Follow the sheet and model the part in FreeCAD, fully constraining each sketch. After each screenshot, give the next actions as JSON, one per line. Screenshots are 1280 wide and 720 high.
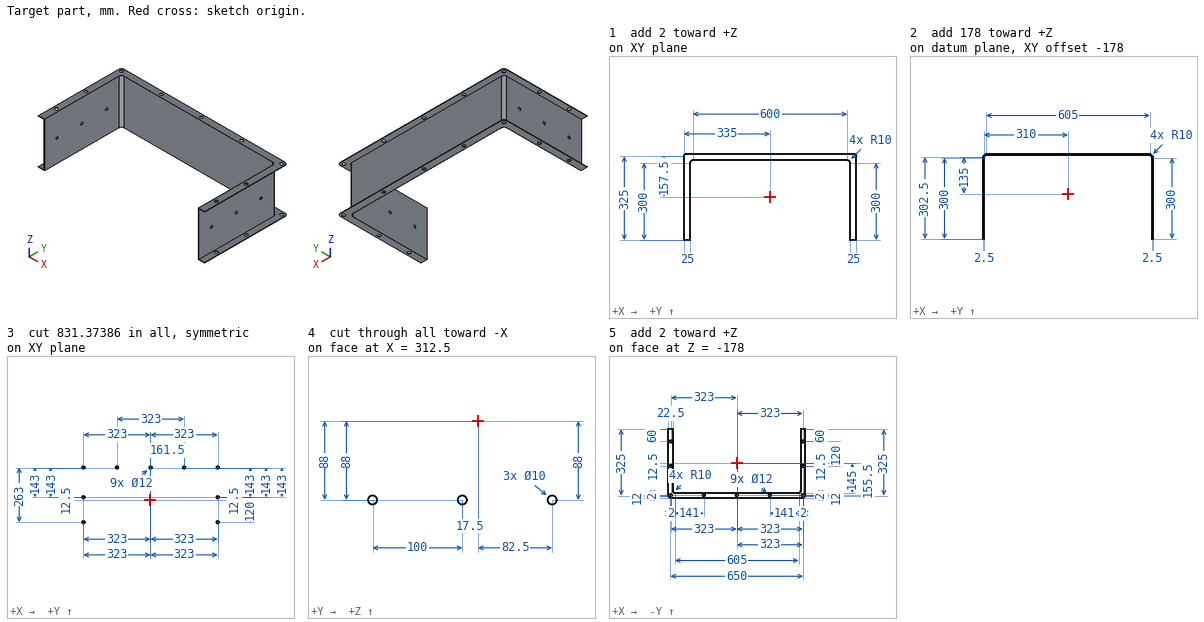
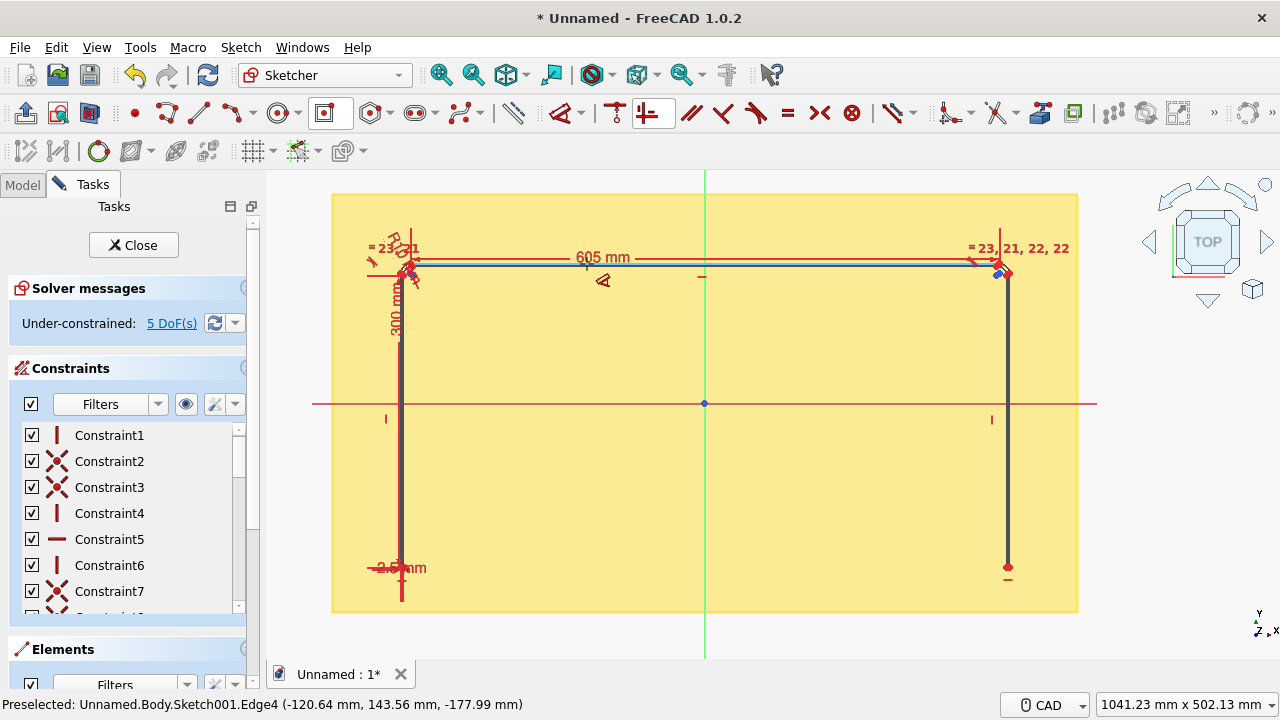
{"action": "scroll", "coordinate": [1008, 568], "scroll_direction": "up", "scroll_amount": 14}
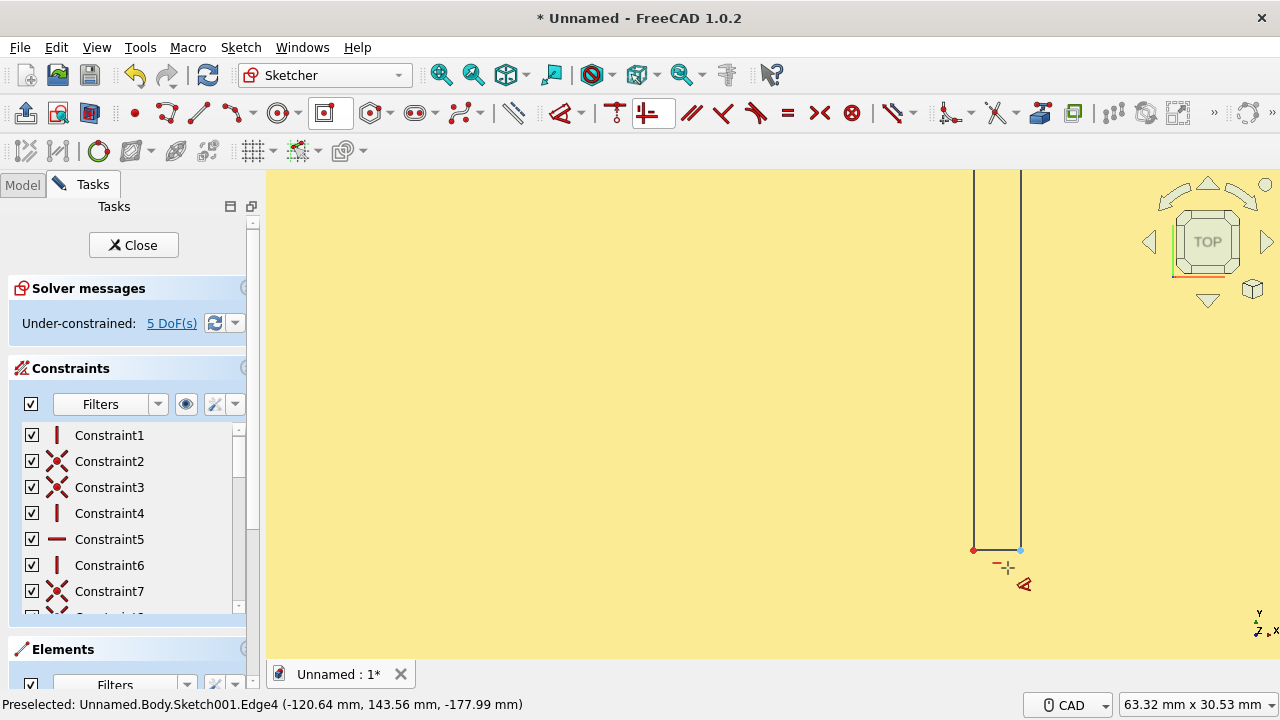
{"action": "left_click", "coordinate": [997, 550]}
{"action": "left_click", "coordinate": [997, 584]}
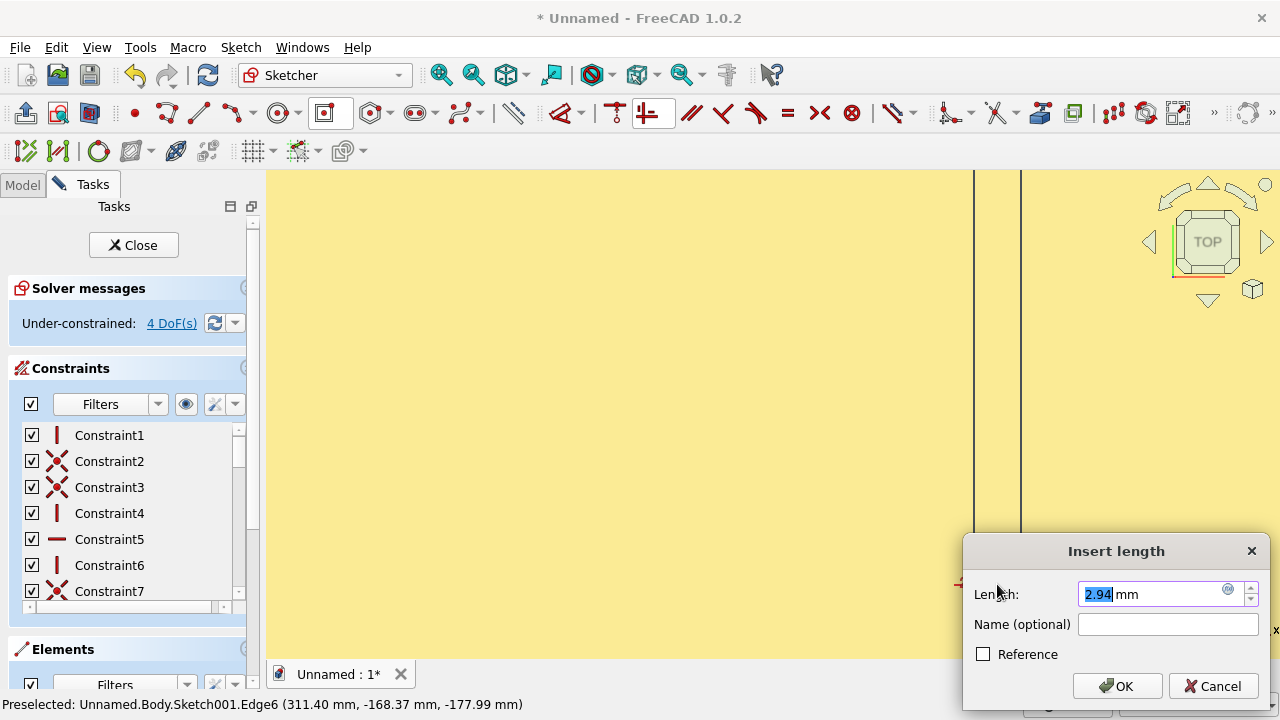
{"action": "type", "text": "2.5"}
{"action": "key", "text": "Return"}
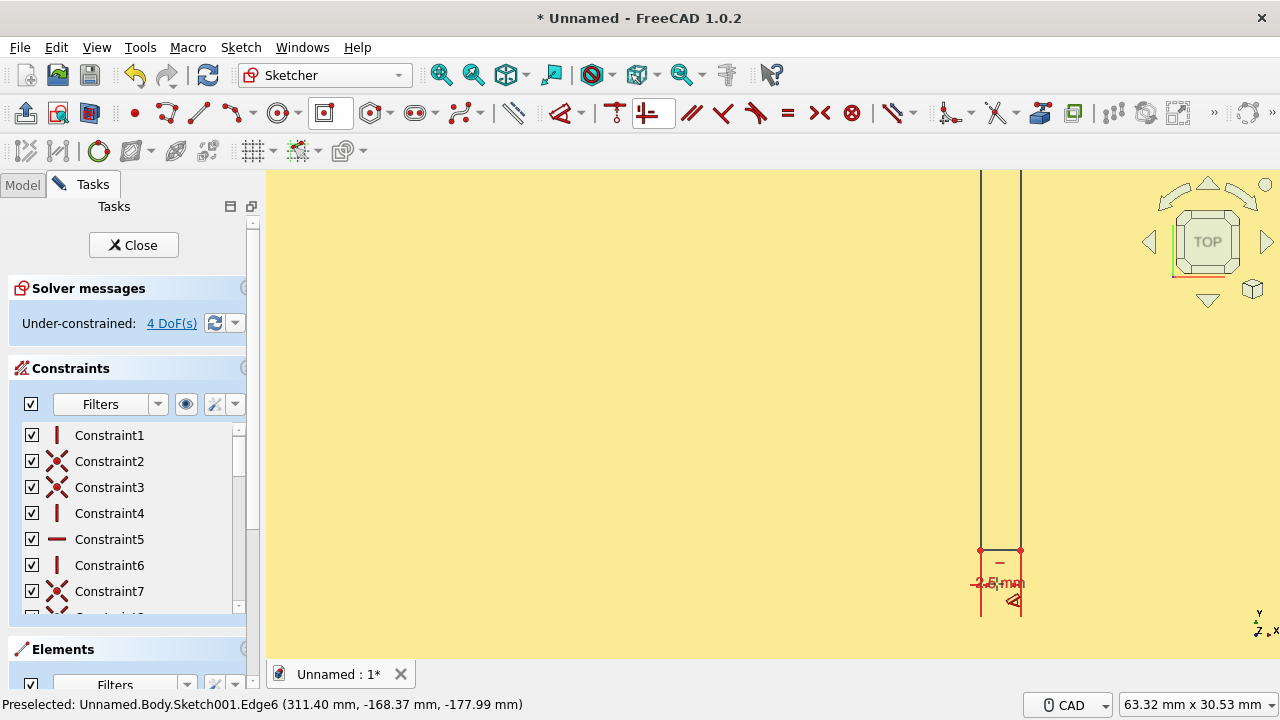
{"action": "scroll", "coordinate": [1008, 569], "scroll_direction": "down", "scroll_amount": 14}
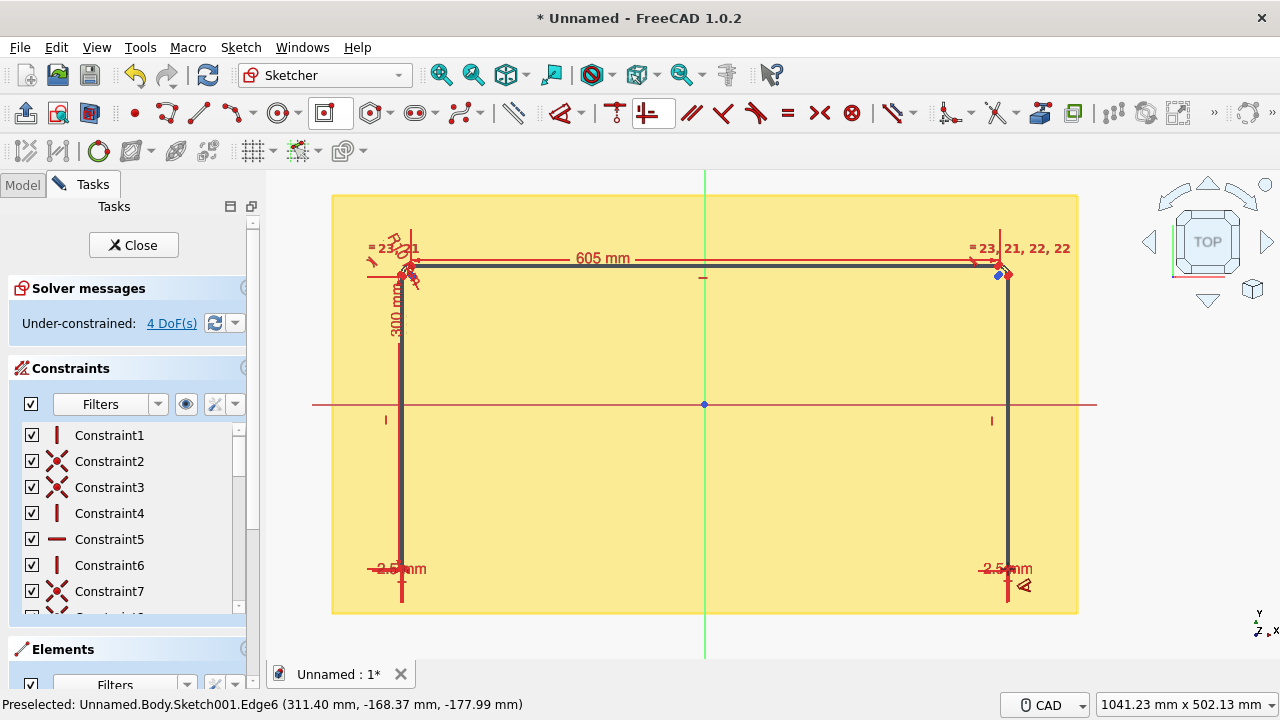
{"action": "scroll", "coordinate": [1007, 481], "scroll_direction": "up", "scroll_amount": 9}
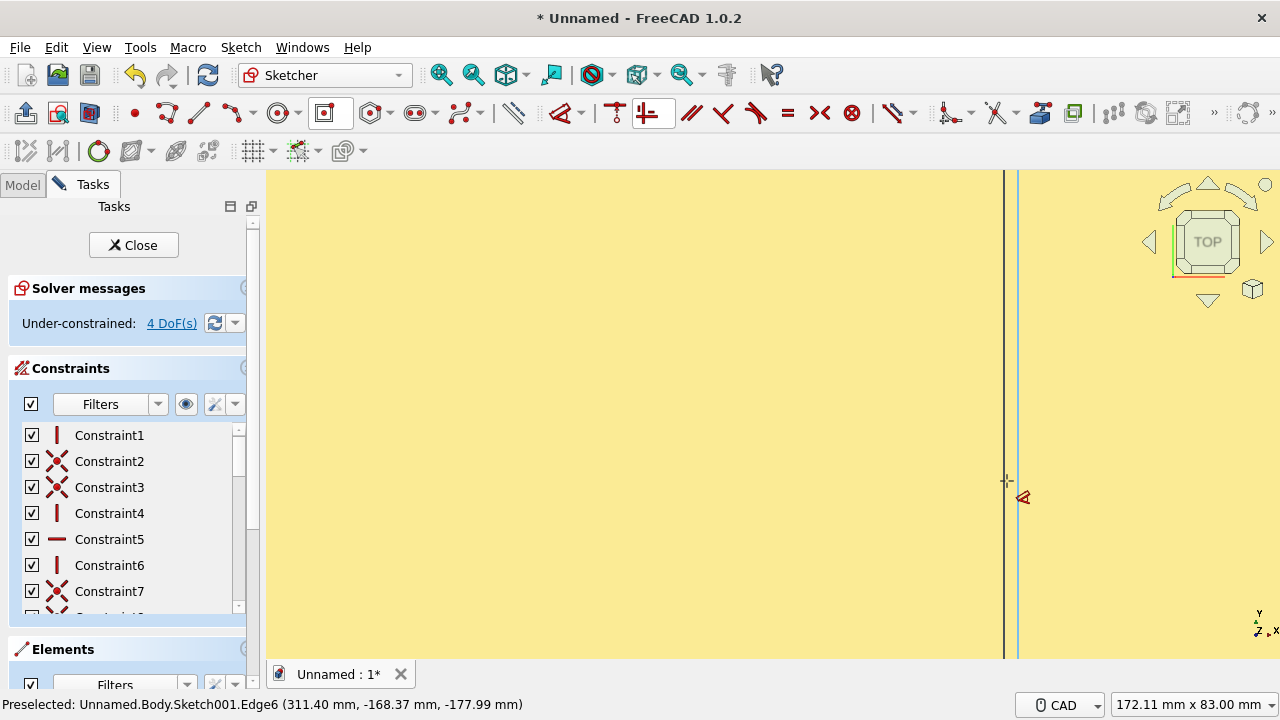
{"action": "left_click", "coordinate": [1004, 478]}
{"action": "left_click", "coordinate": [1038, 414]}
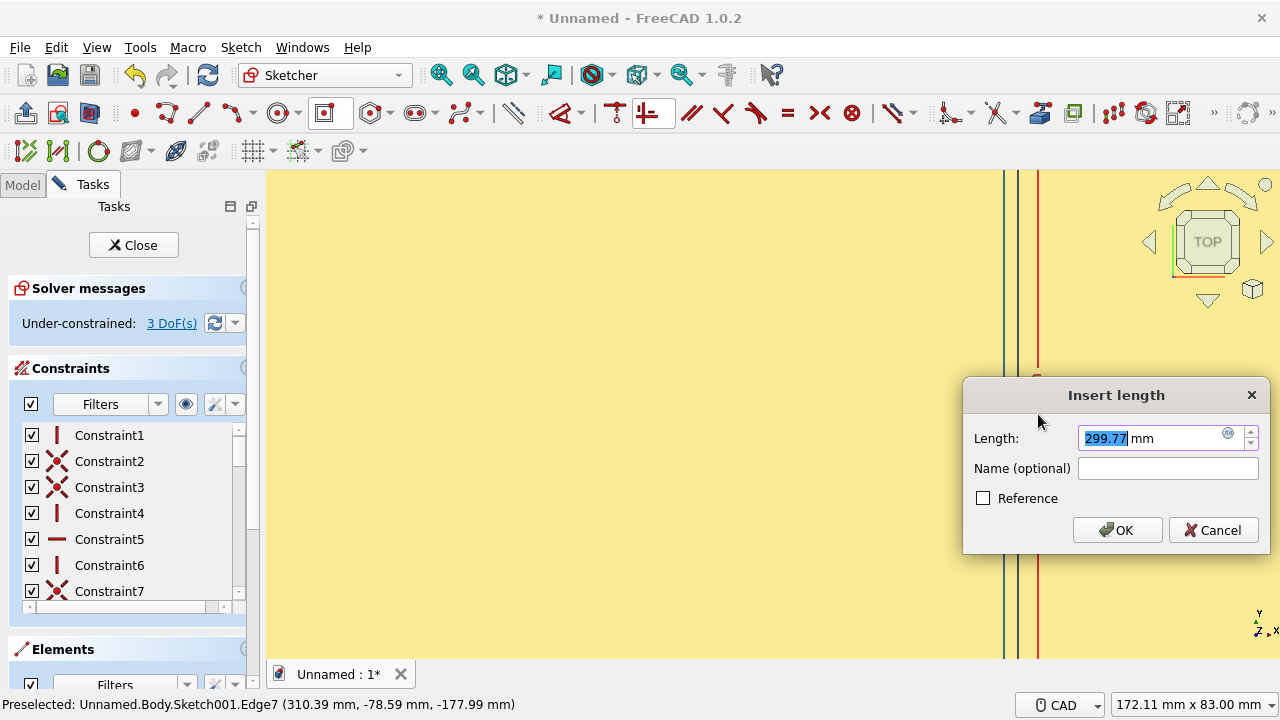
{"action": "type", "text": "300"}
{"action": "key", "text": "Return"}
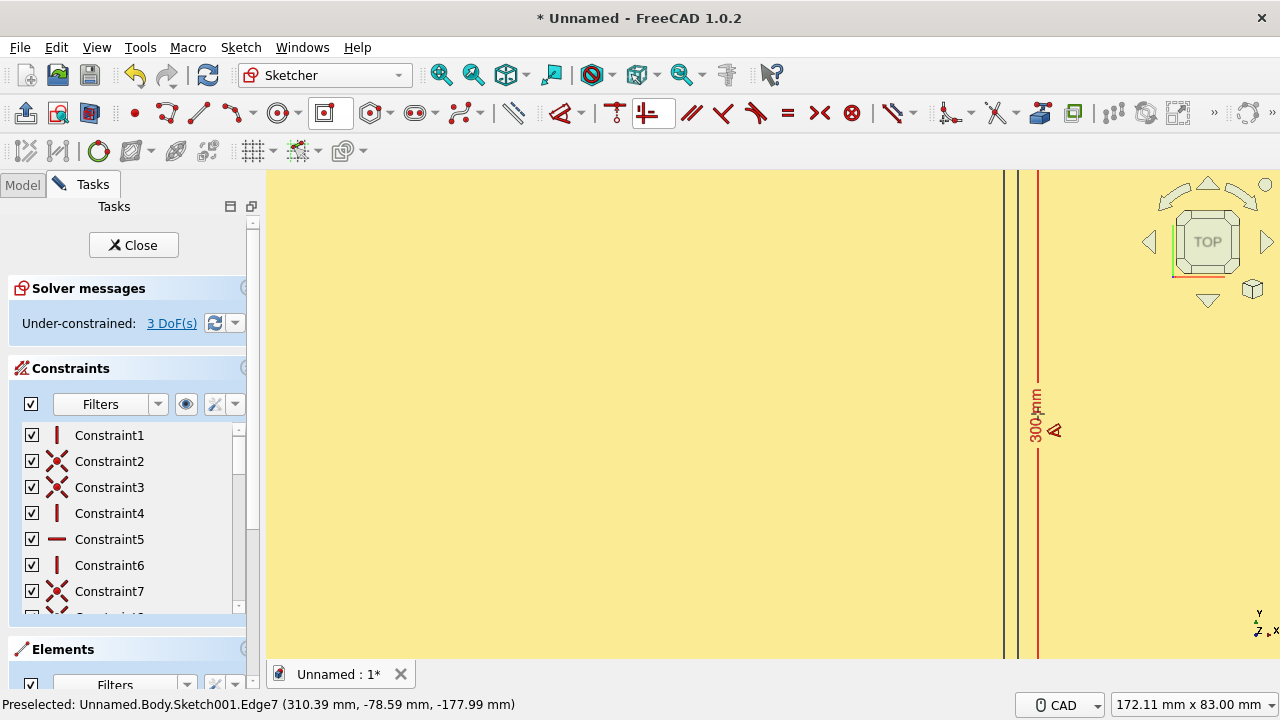
{"action": "scroll", "coordinate": [1007, 480], "scroll_direction": "down", "scroll_amount": 9}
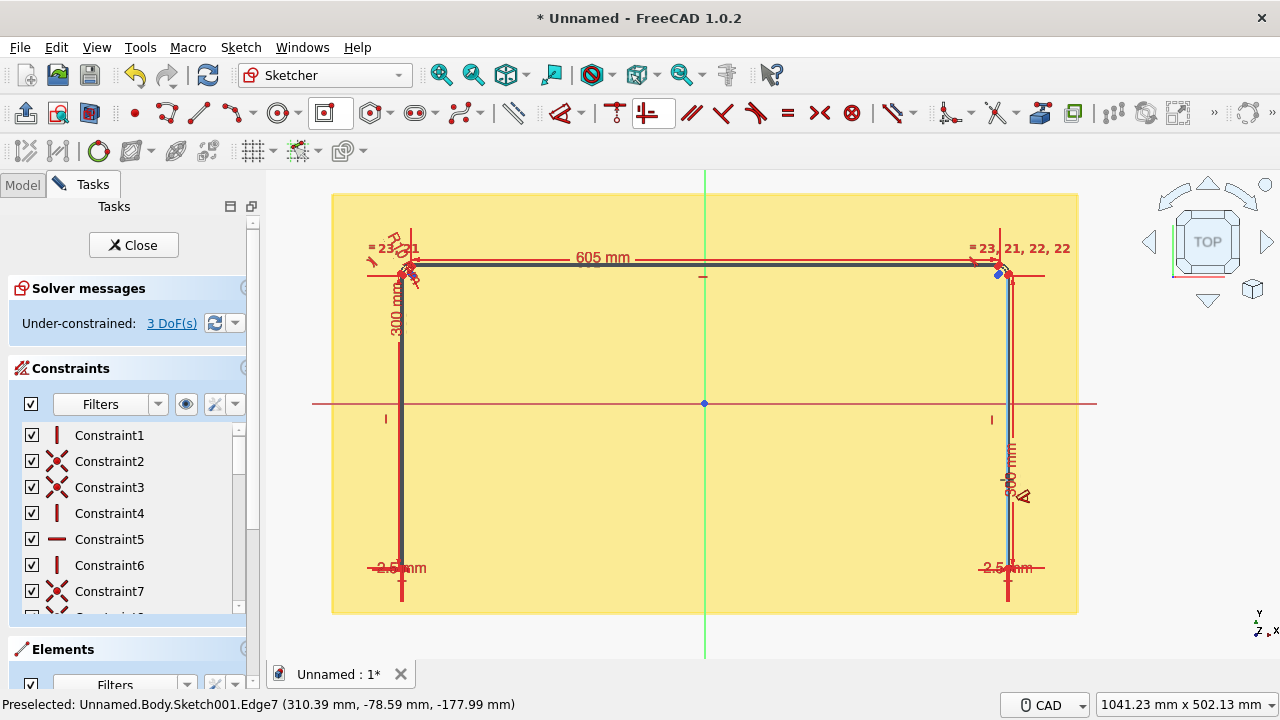
{"action": "scroll", "coordinate": [403, 276], "scroll_direction": "up", "scroll_amount": 7}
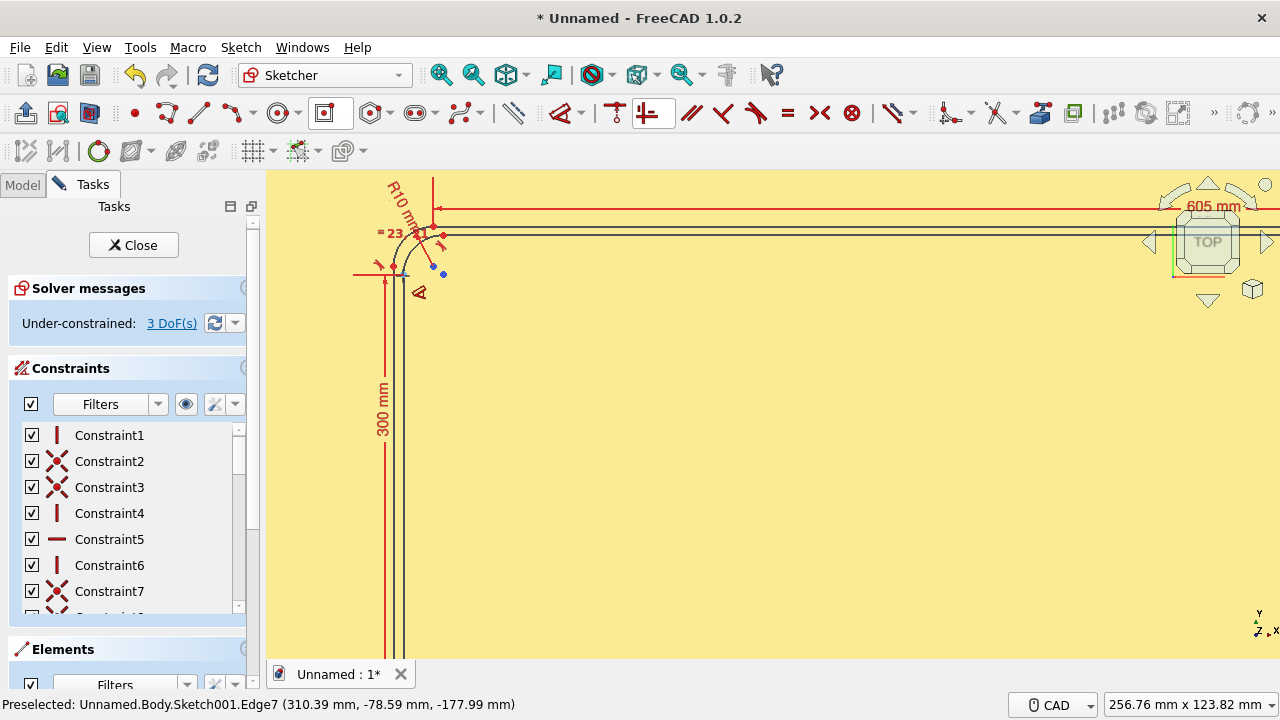
{"action": "left_click", "coordinate": [404, 275]}
{"action": "left_click", "coordinate": [759, 217]}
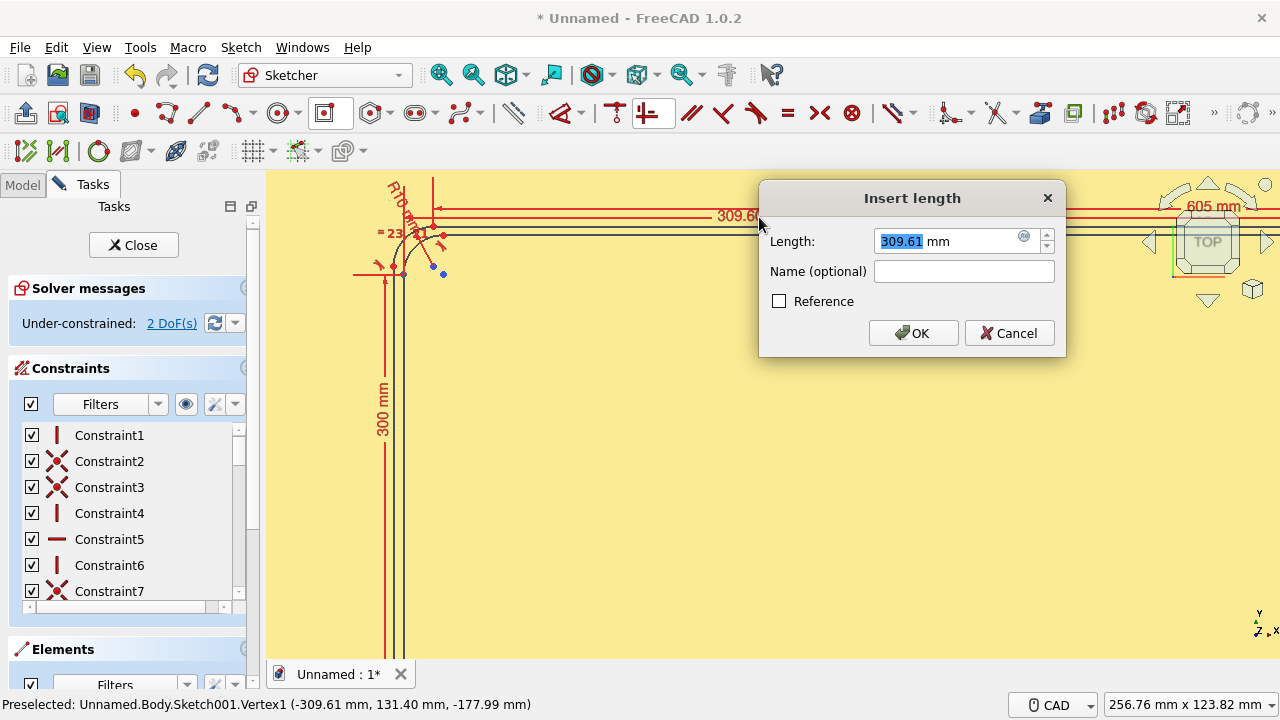
{"action": "type", "text": "310"}
{"action": "key", "text": "Return"}